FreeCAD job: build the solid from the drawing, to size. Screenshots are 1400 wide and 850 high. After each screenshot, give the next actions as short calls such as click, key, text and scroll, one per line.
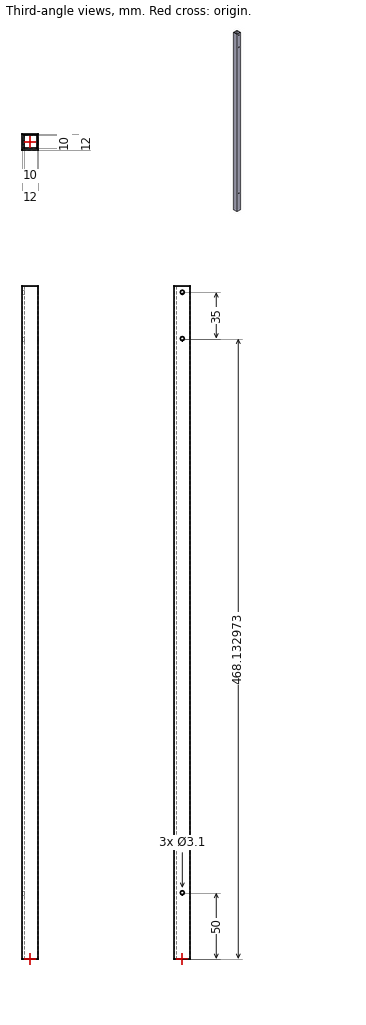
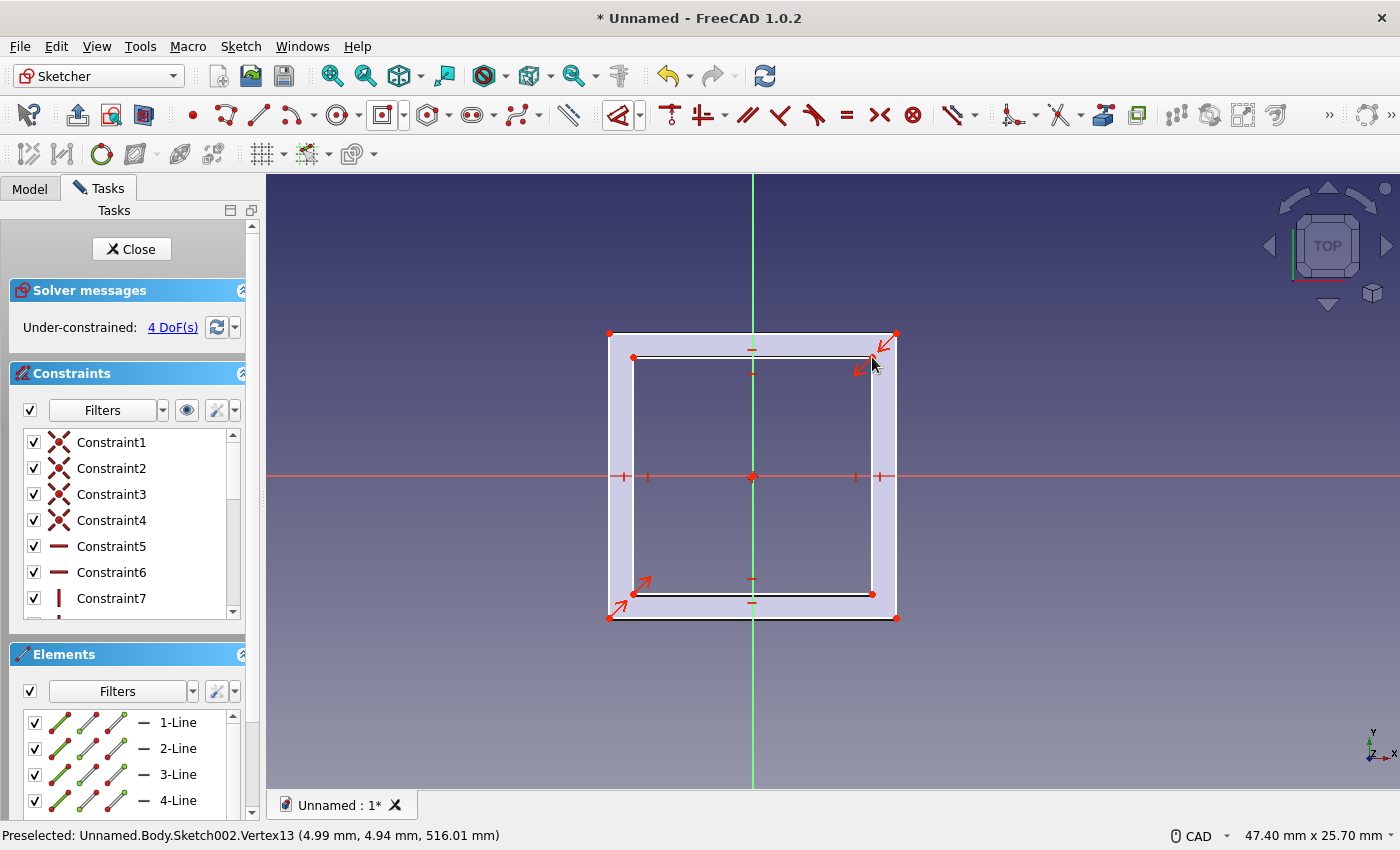
click(695, 618)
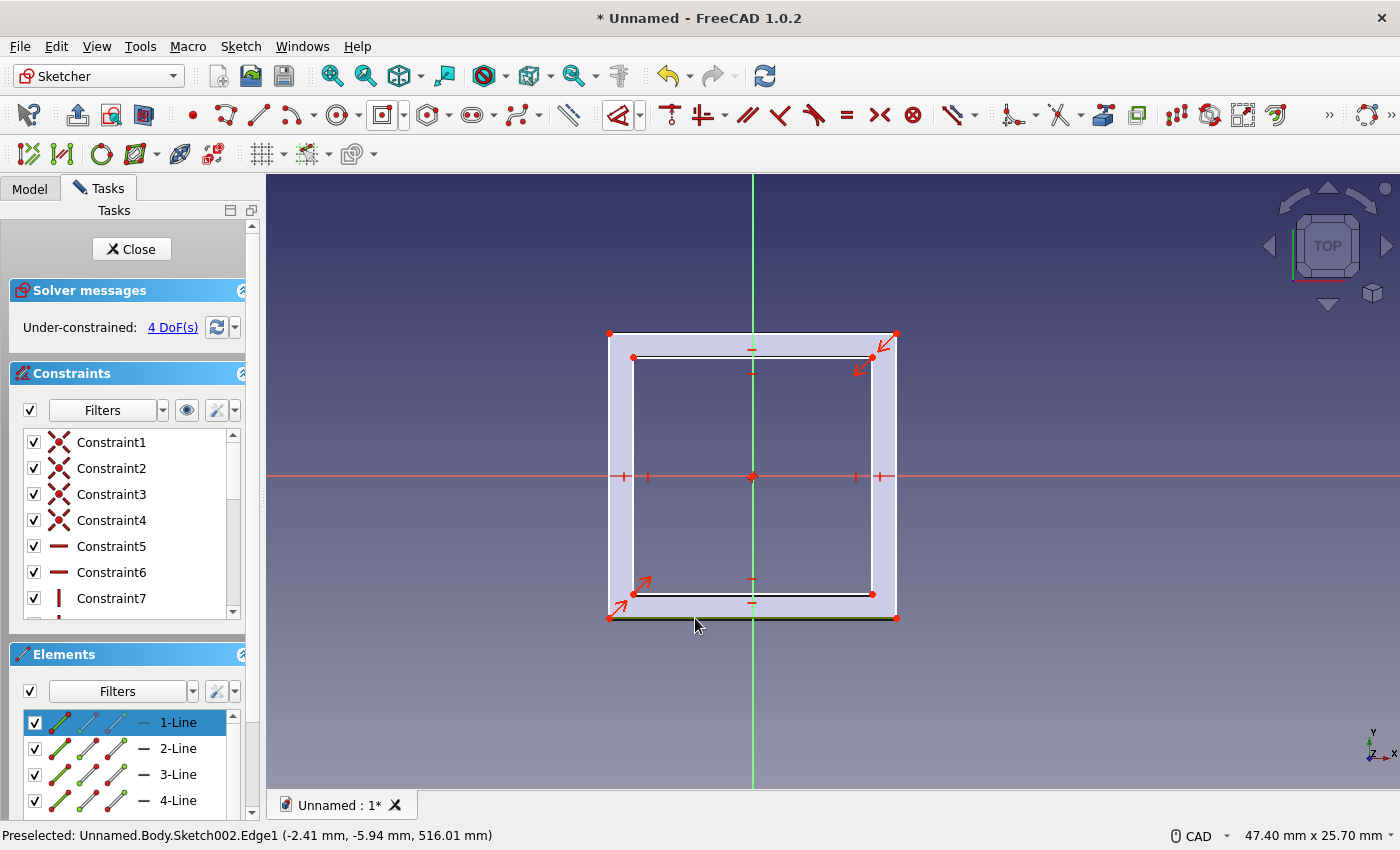
key(l)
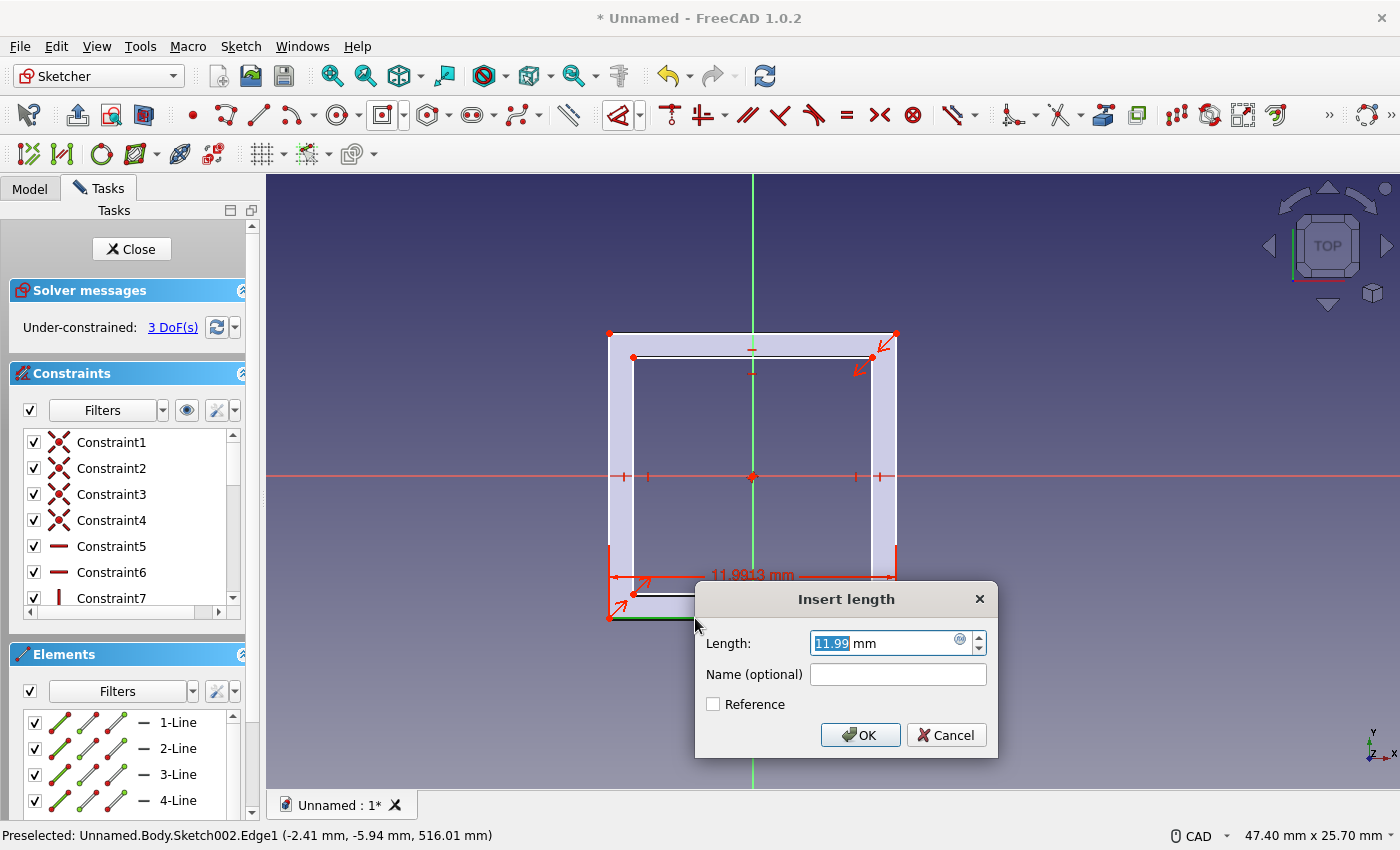
text(12)
key(Return)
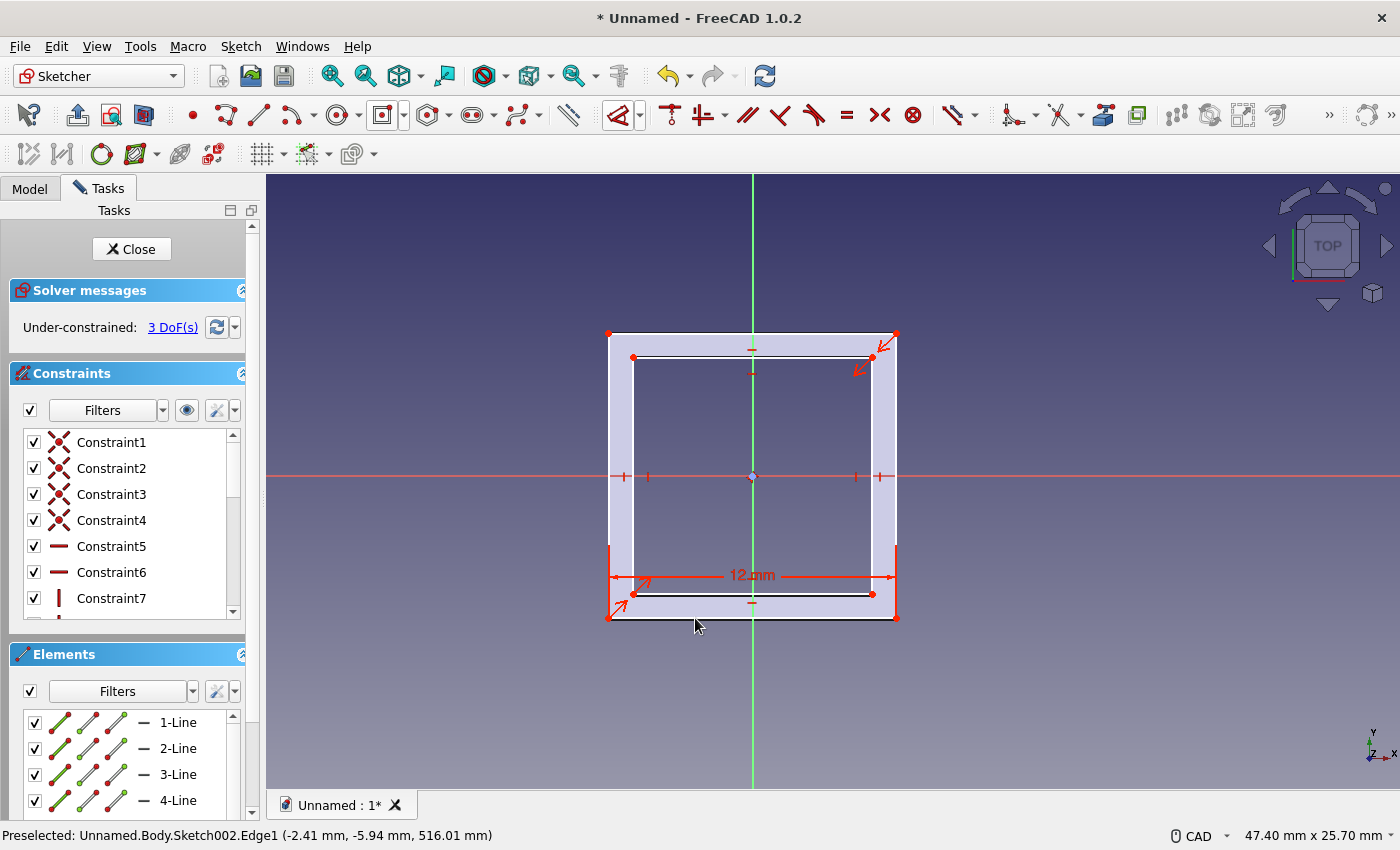
click(896, 533)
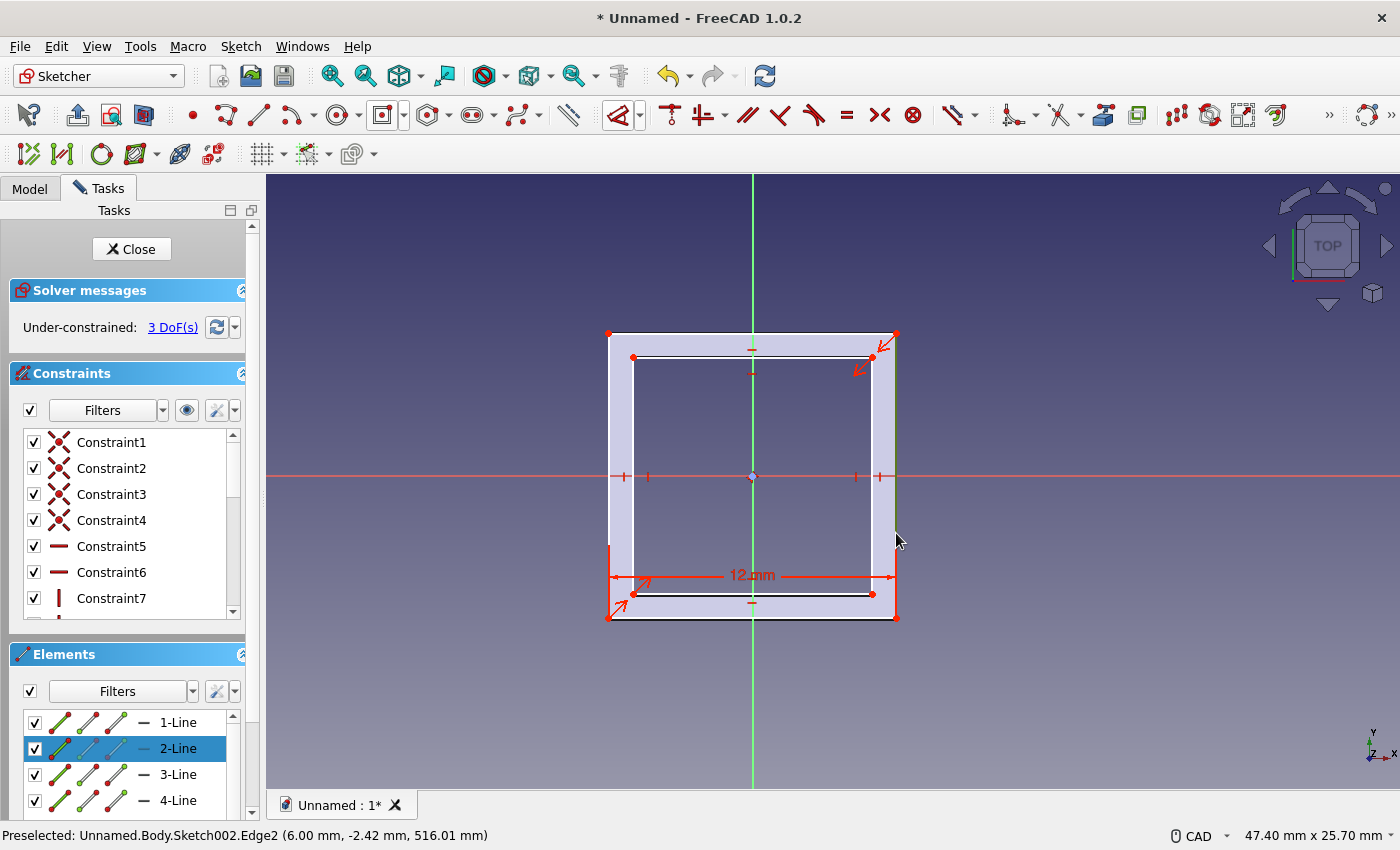
key(i)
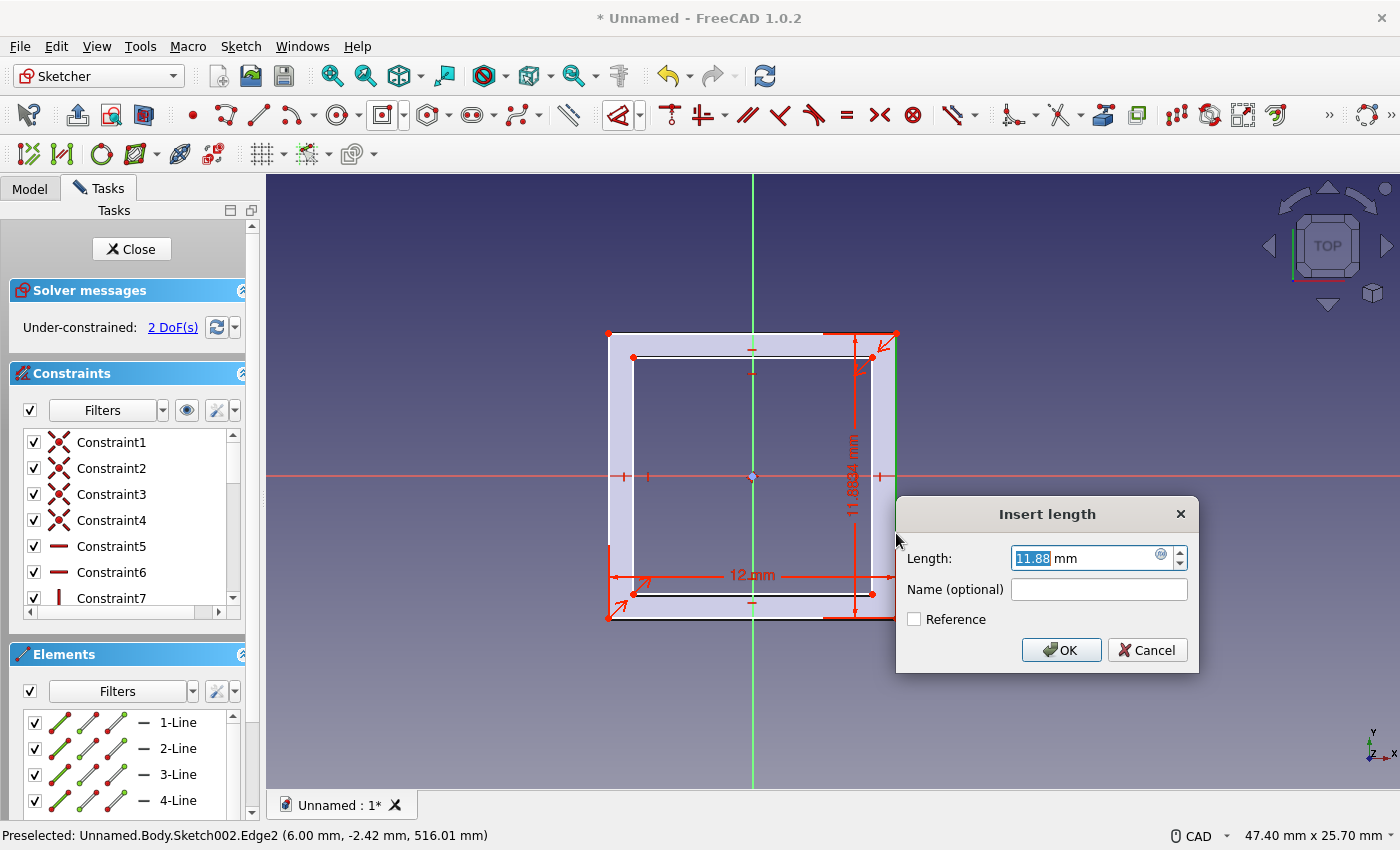
text(12)
key(Return)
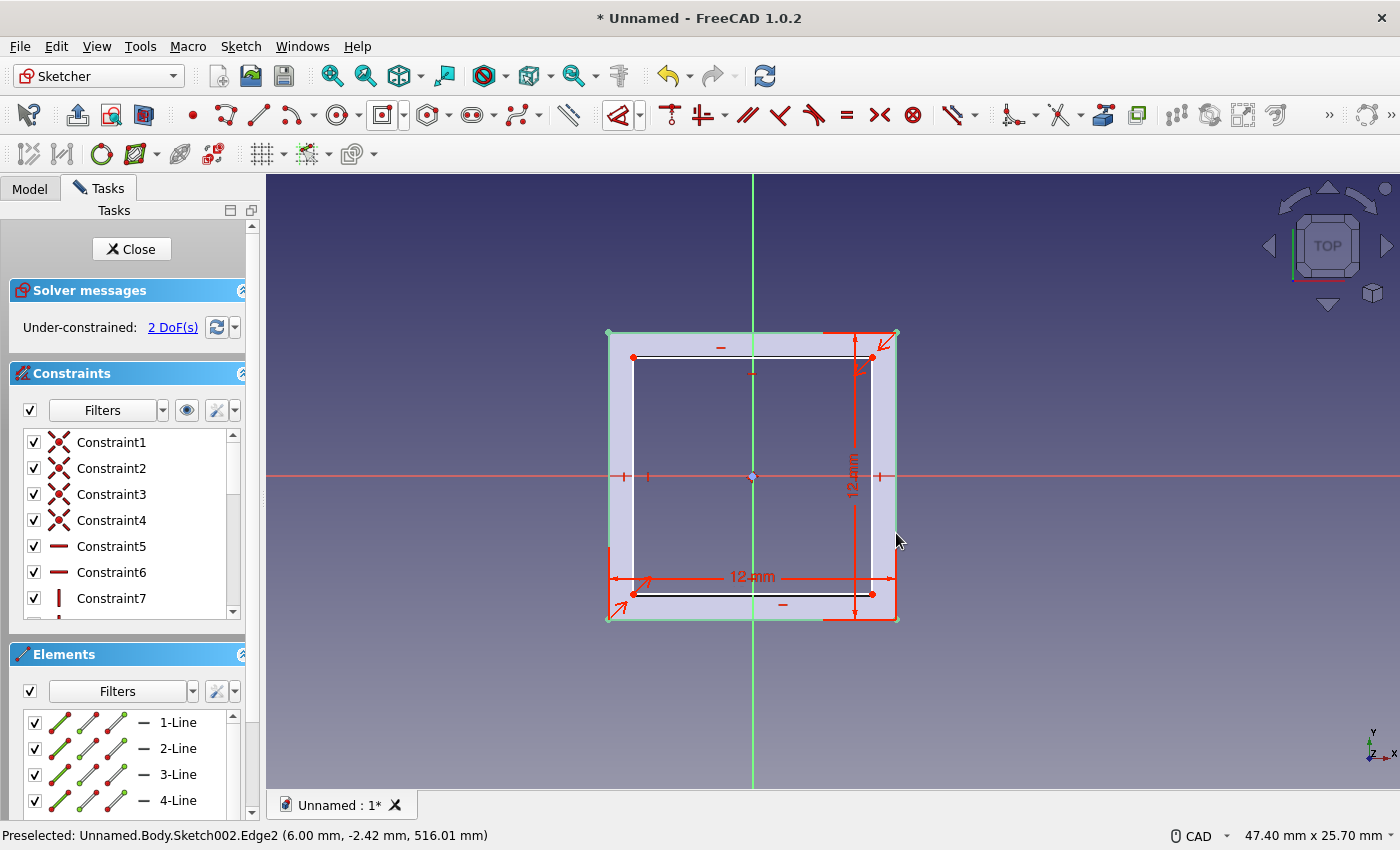
click(705, 594)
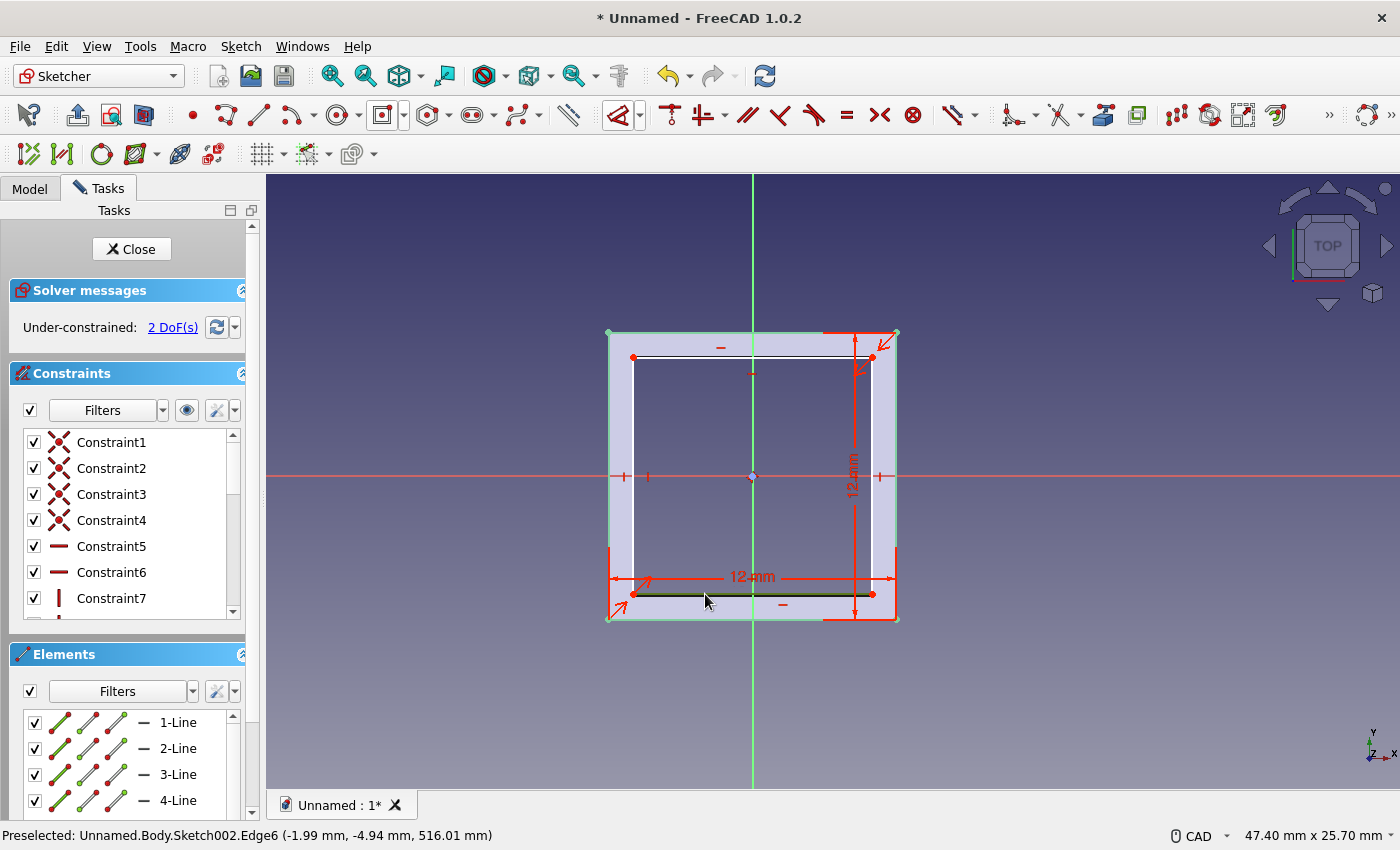
click(640, 116)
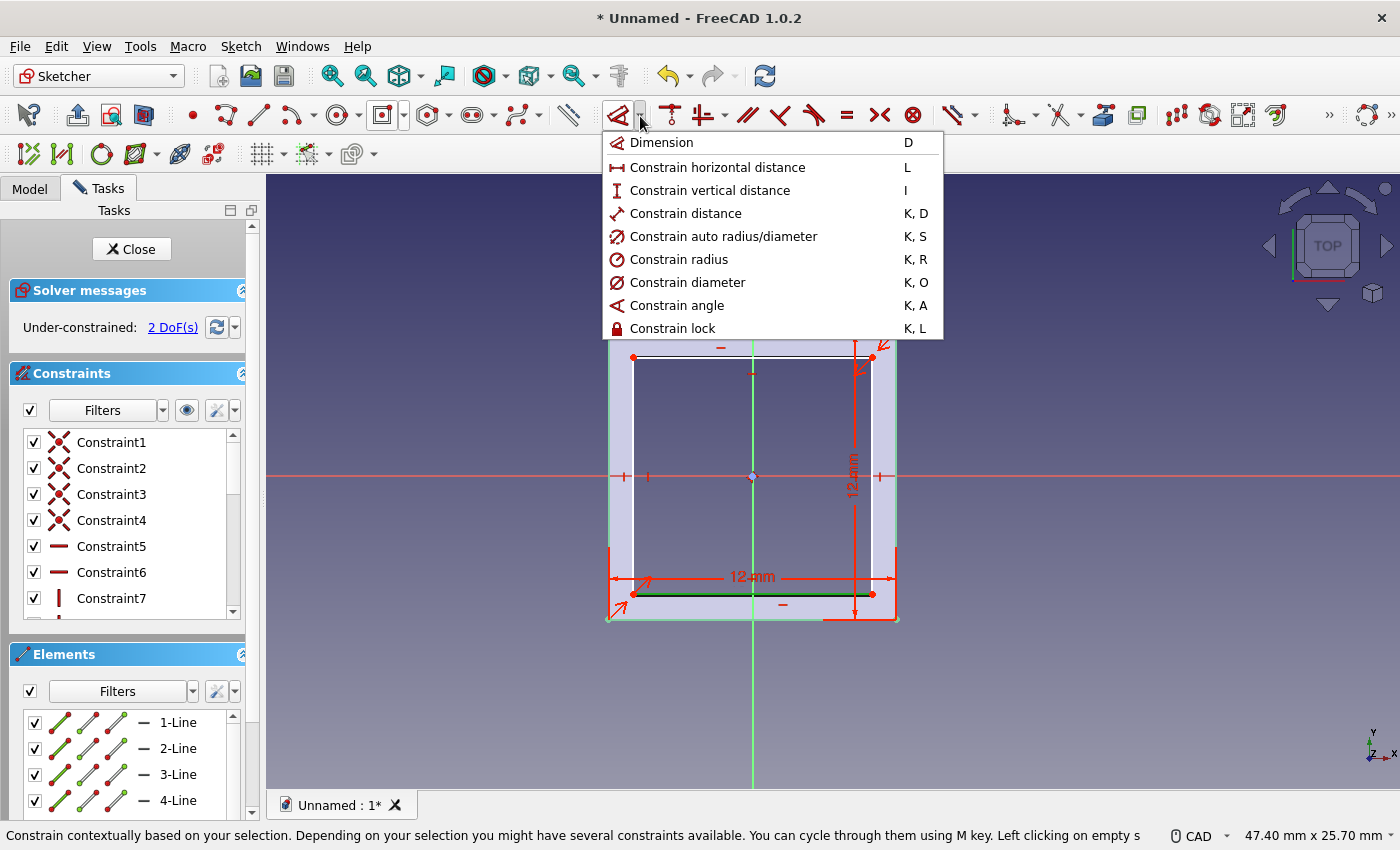
click(773, 168)